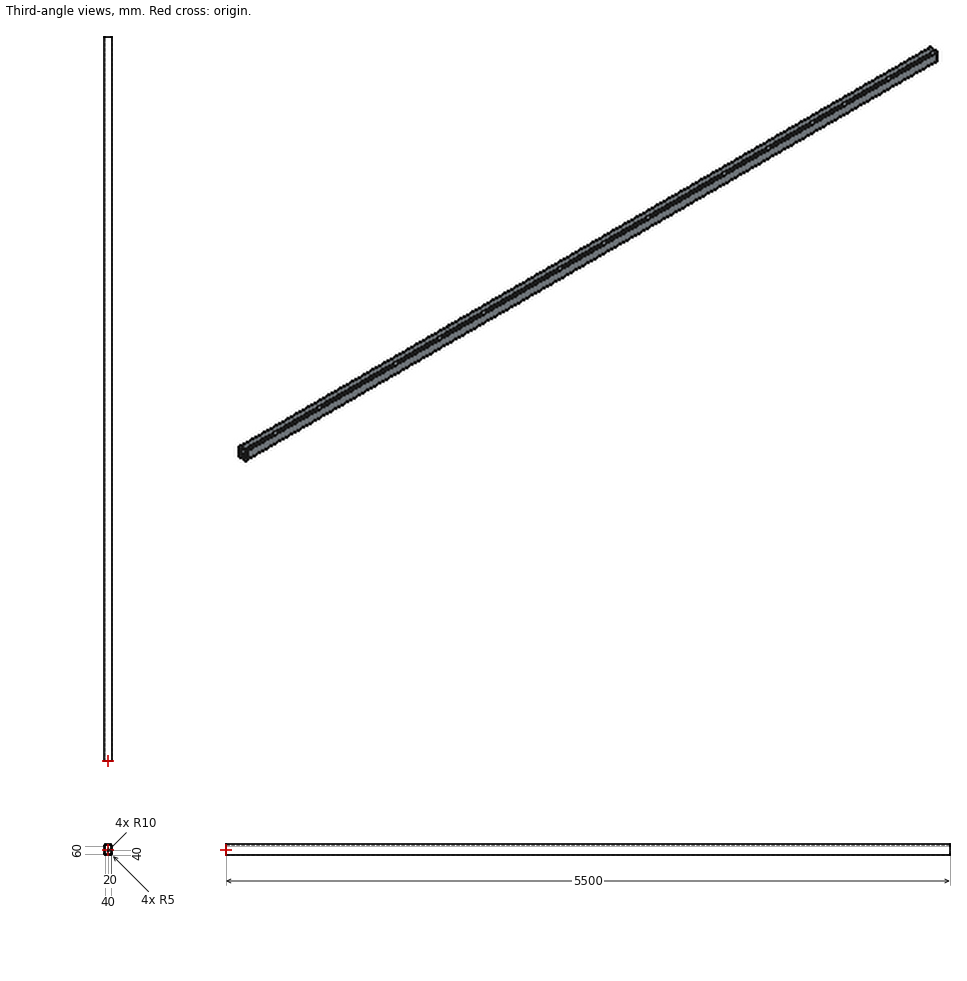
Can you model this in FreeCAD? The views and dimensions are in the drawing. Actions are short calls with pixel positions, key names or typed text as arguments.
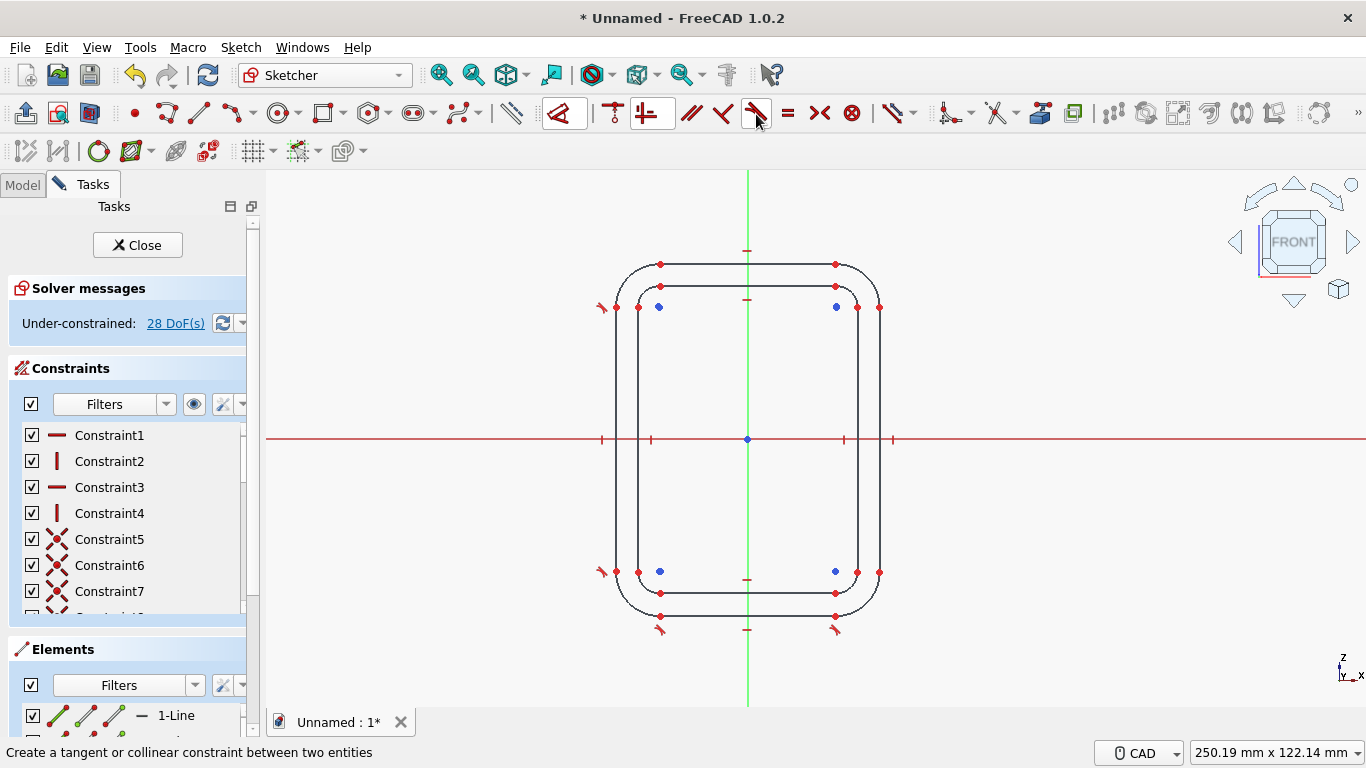
click(713, 264)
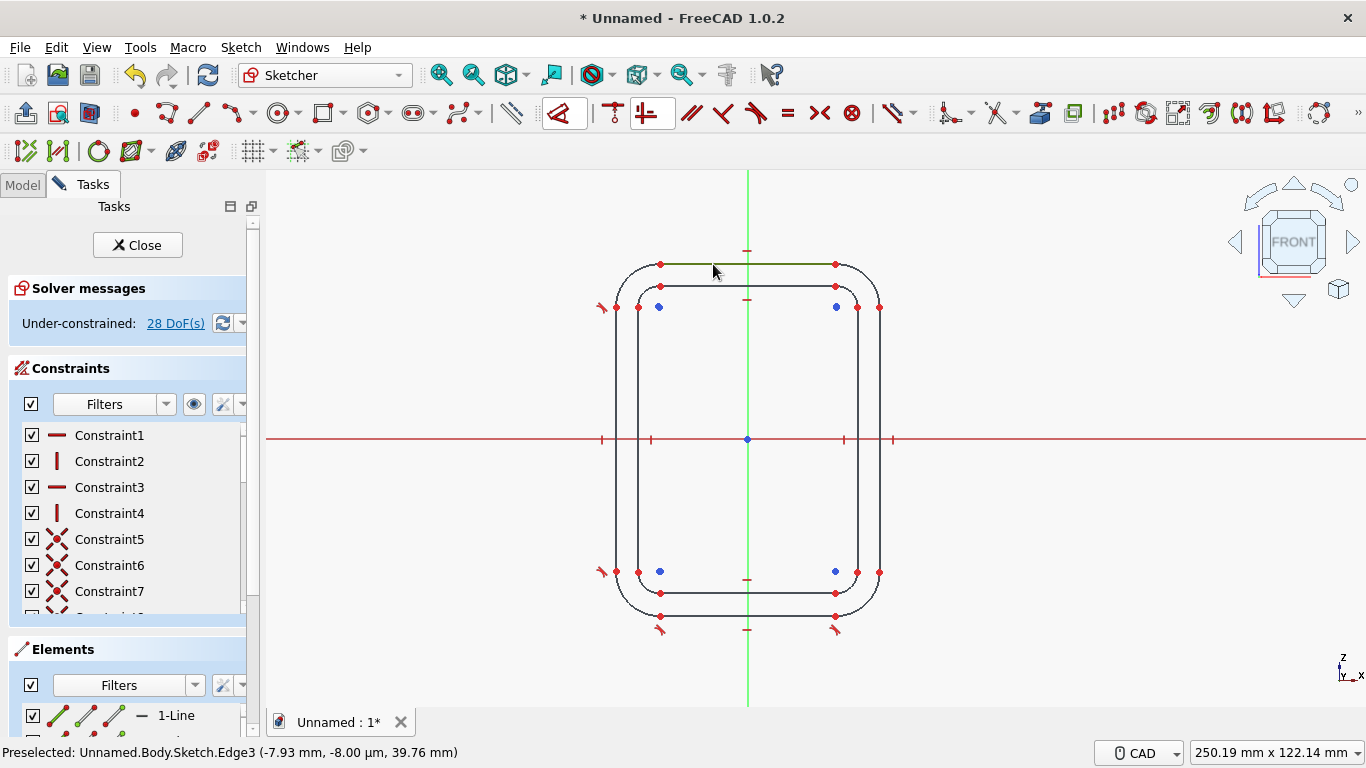
click(640, 269)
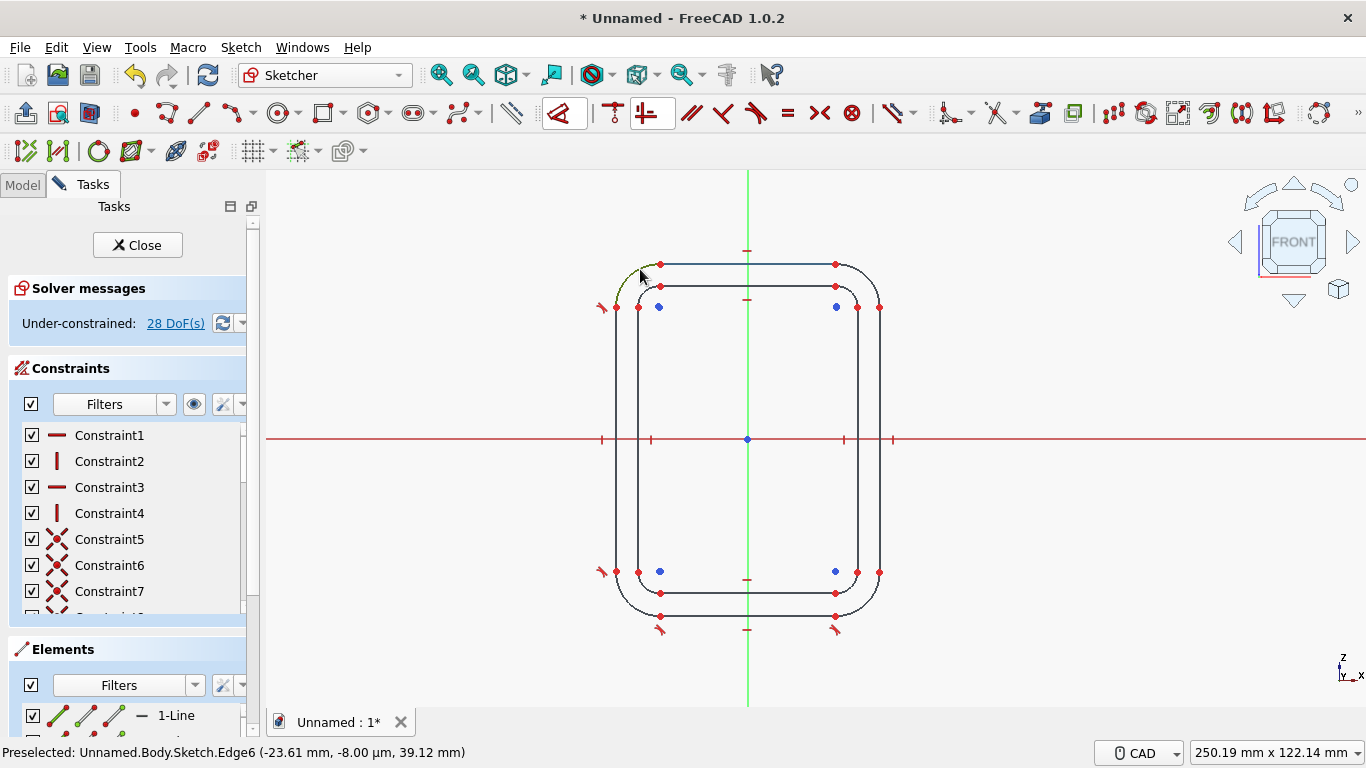
click(756, 114)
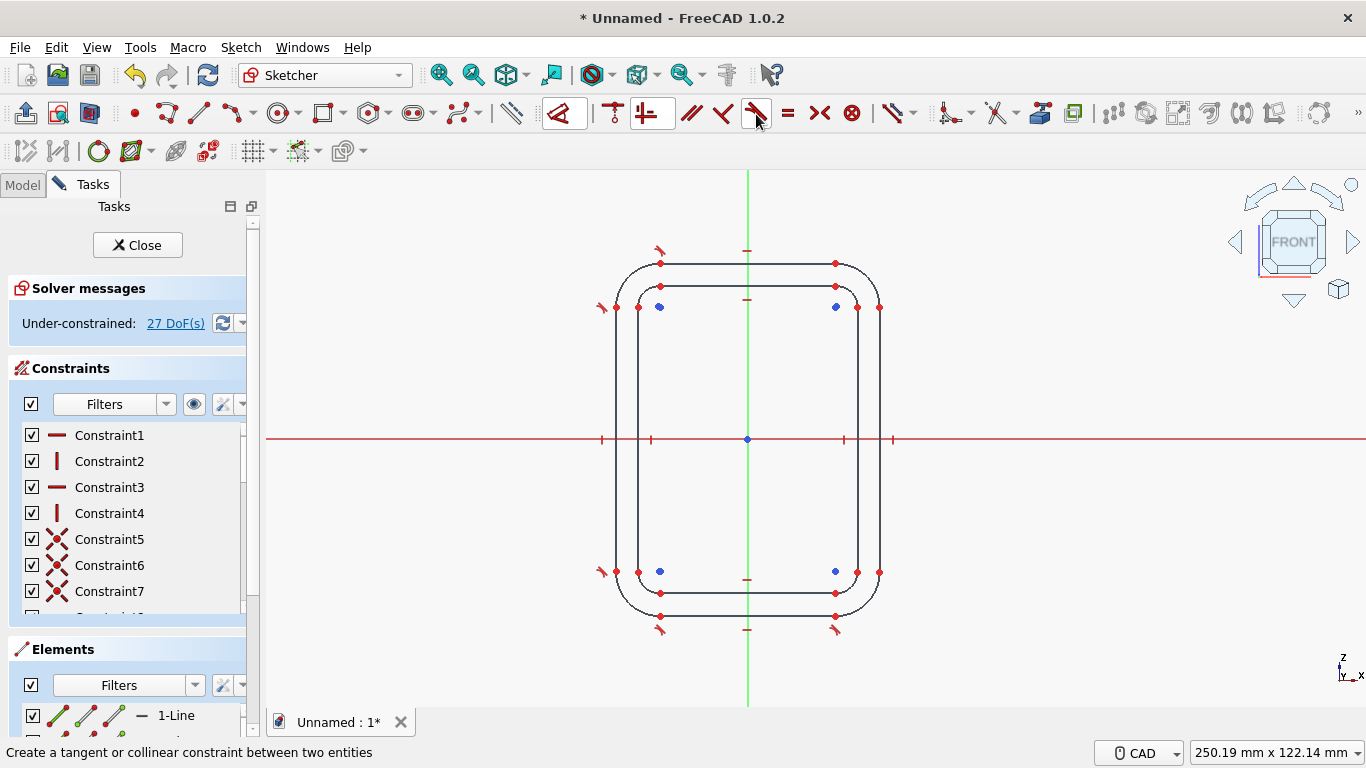
click(713, 264)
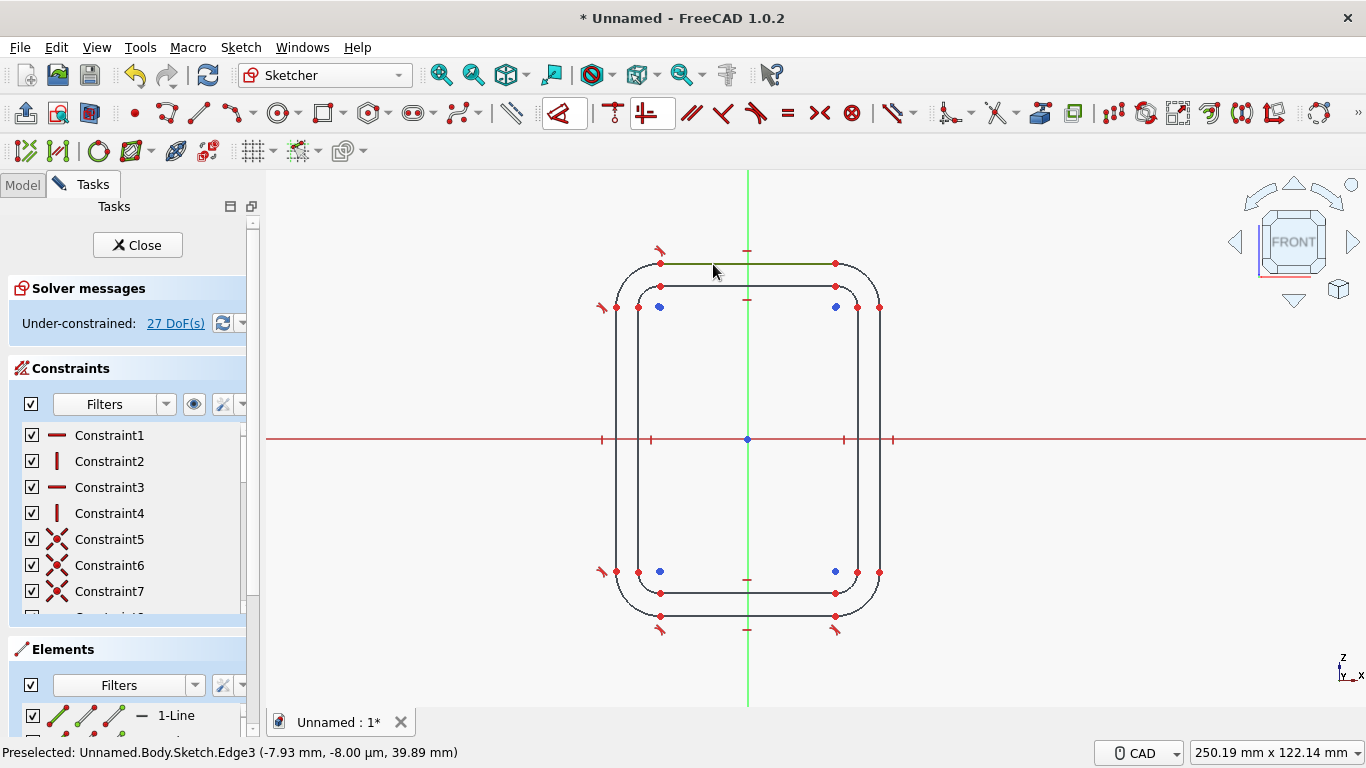
click(875, 288)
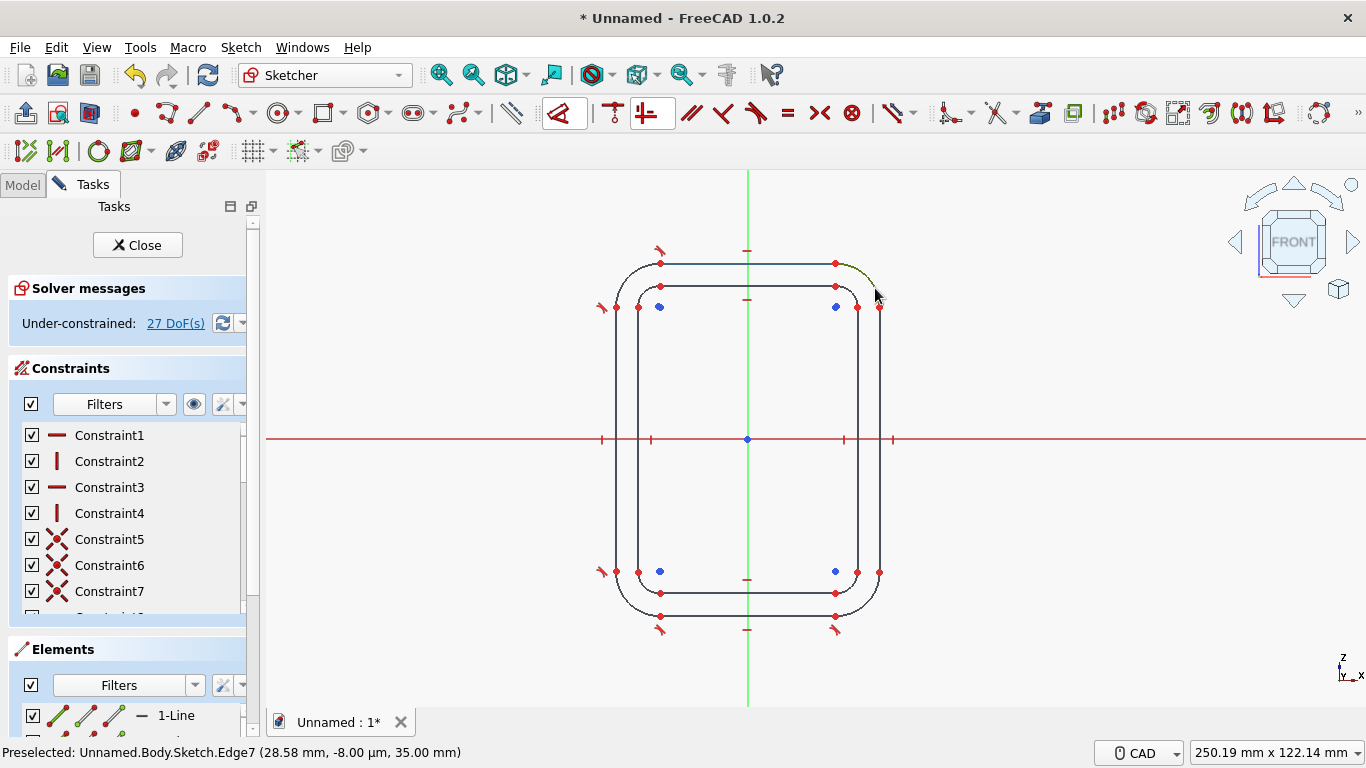
click(756, 114)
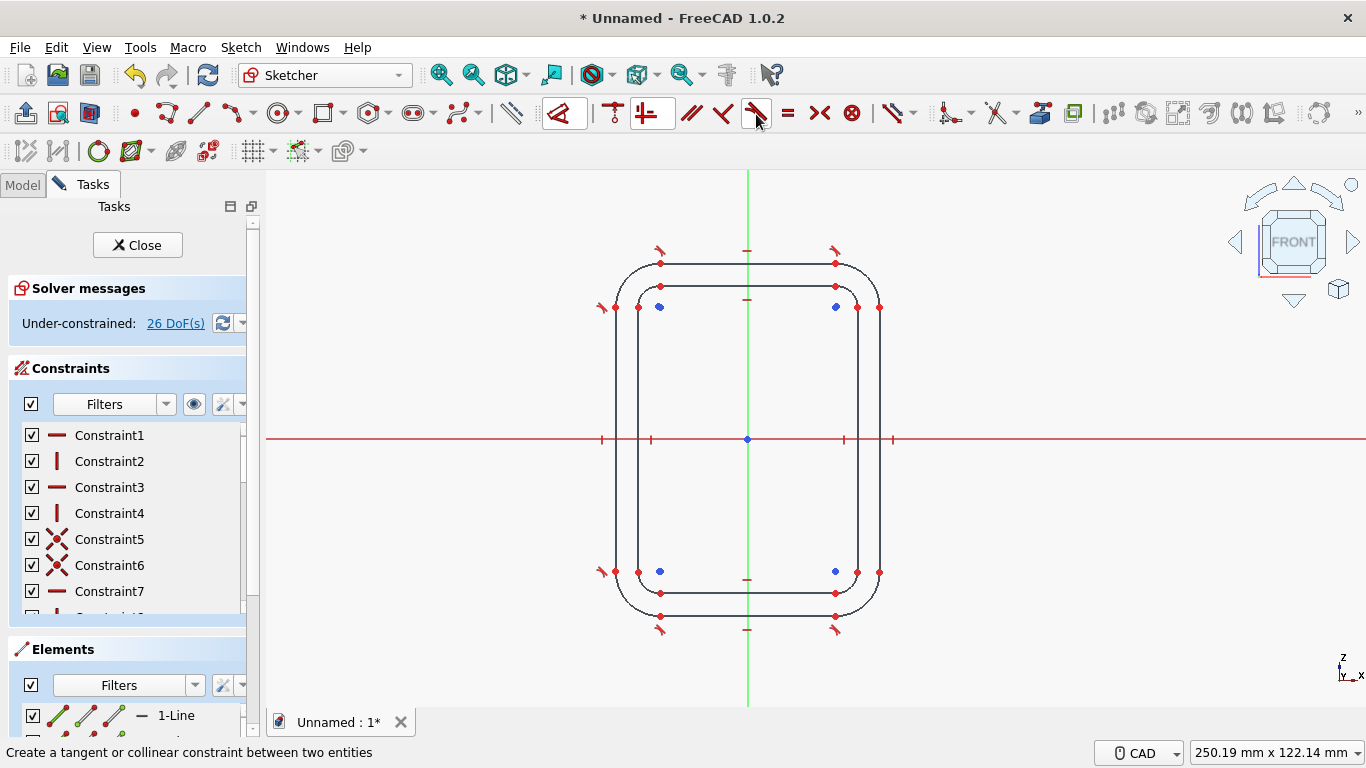
click(880, 387)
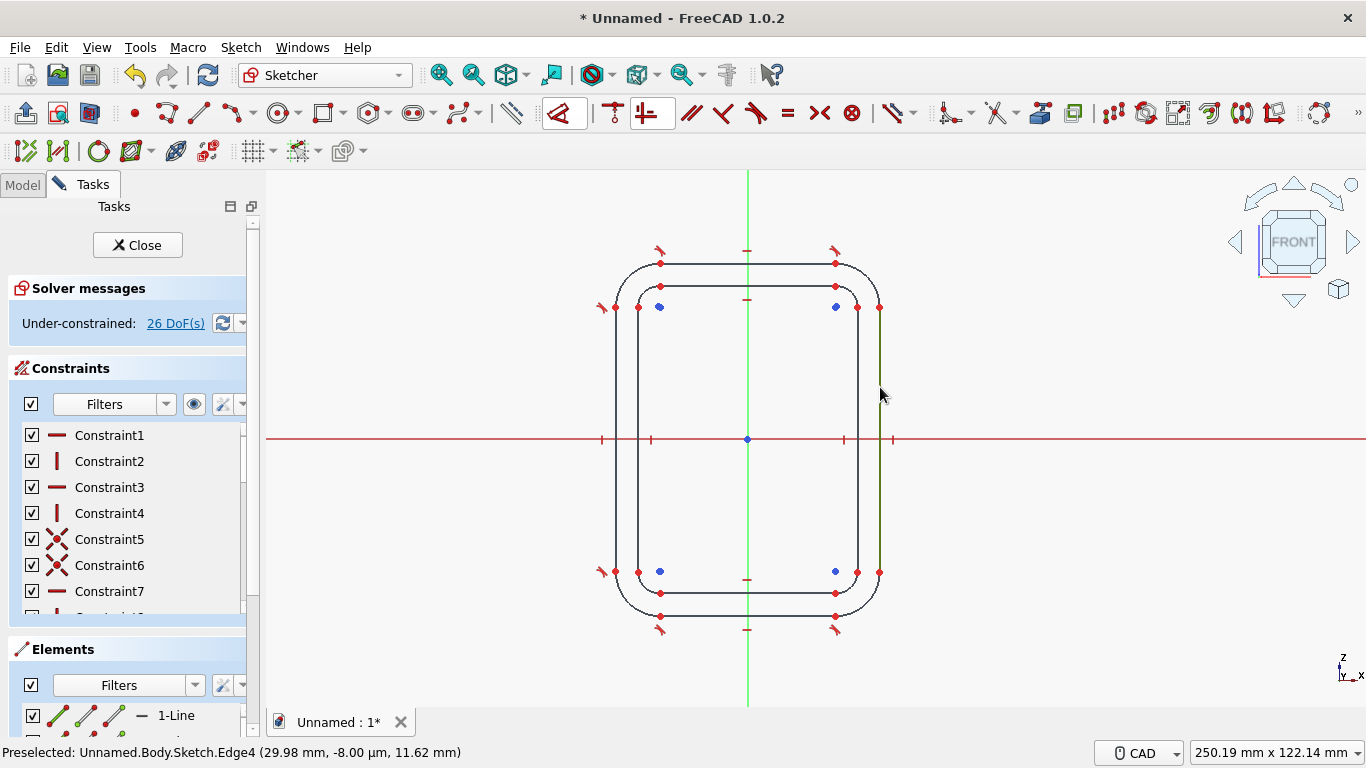
click(875, 288)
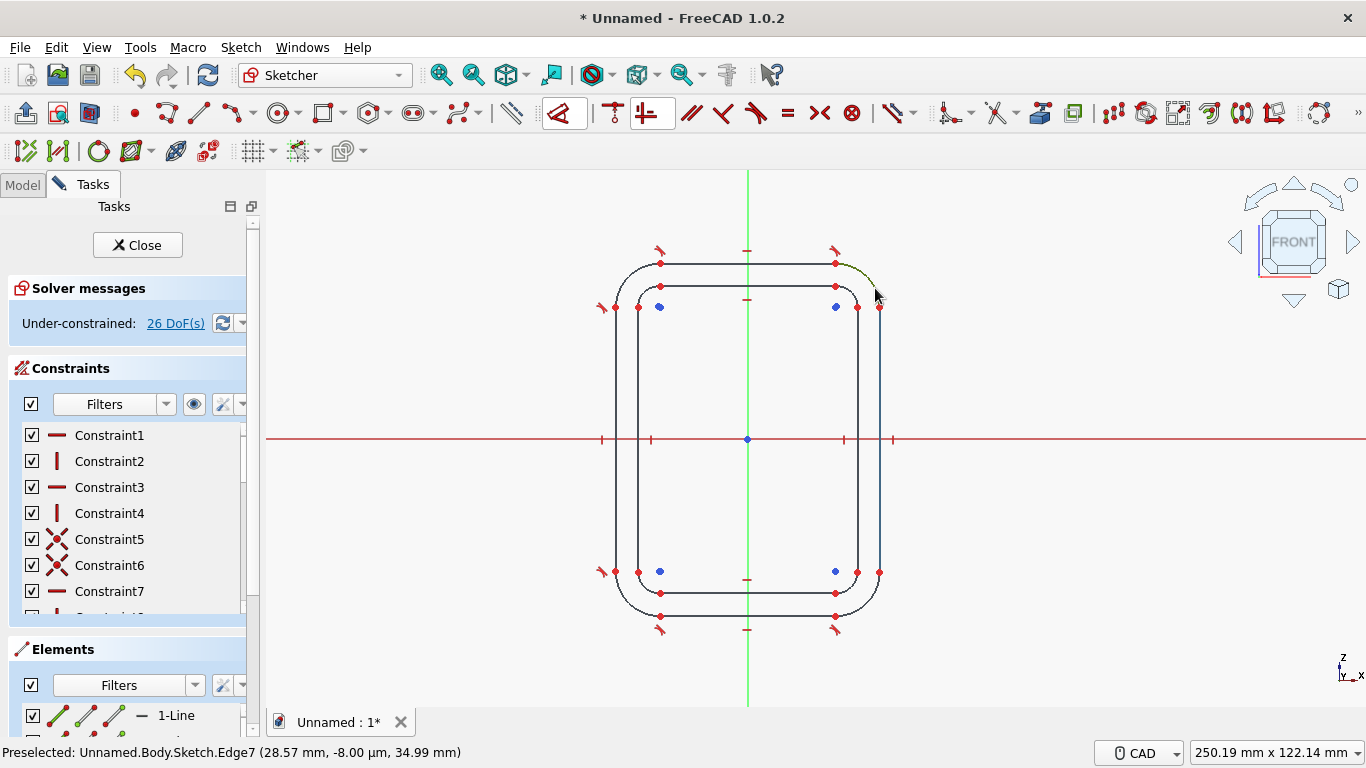
click(756, 114)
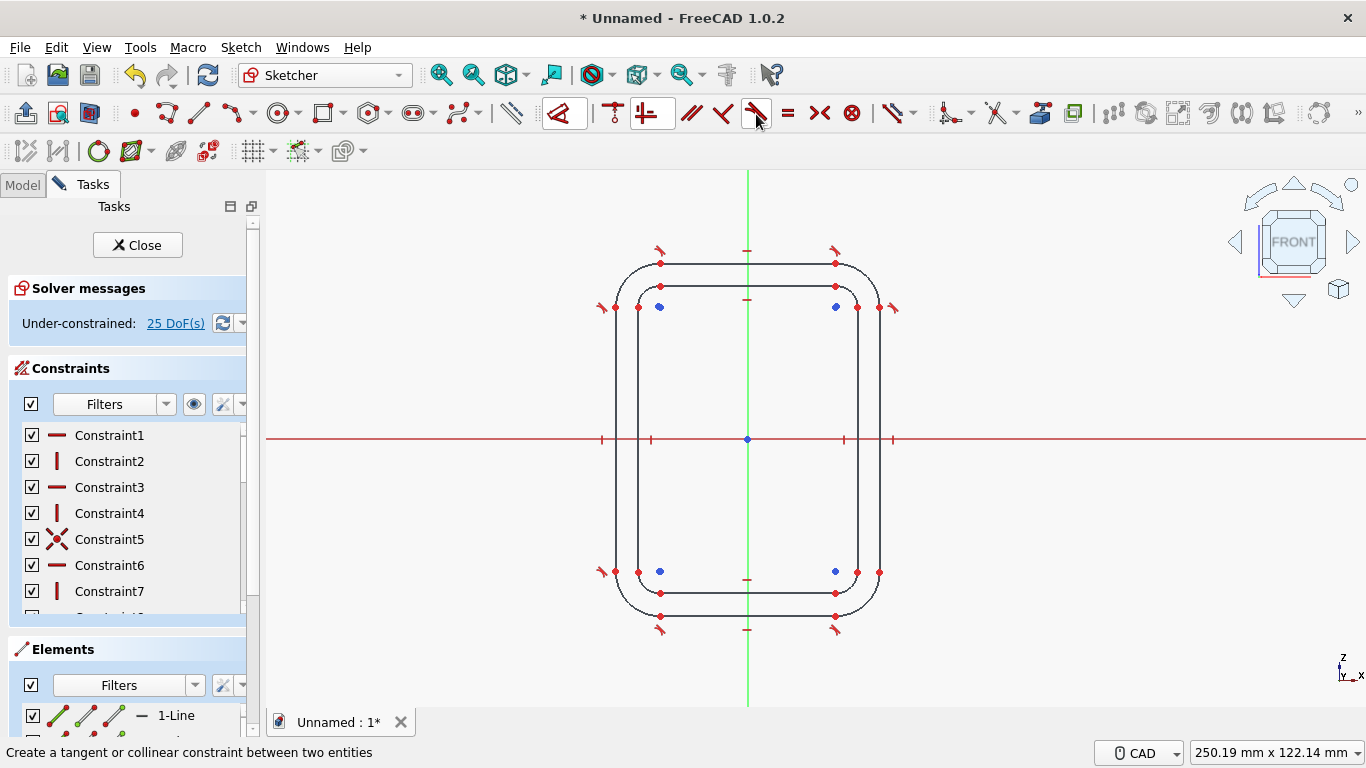
click(880, 387)